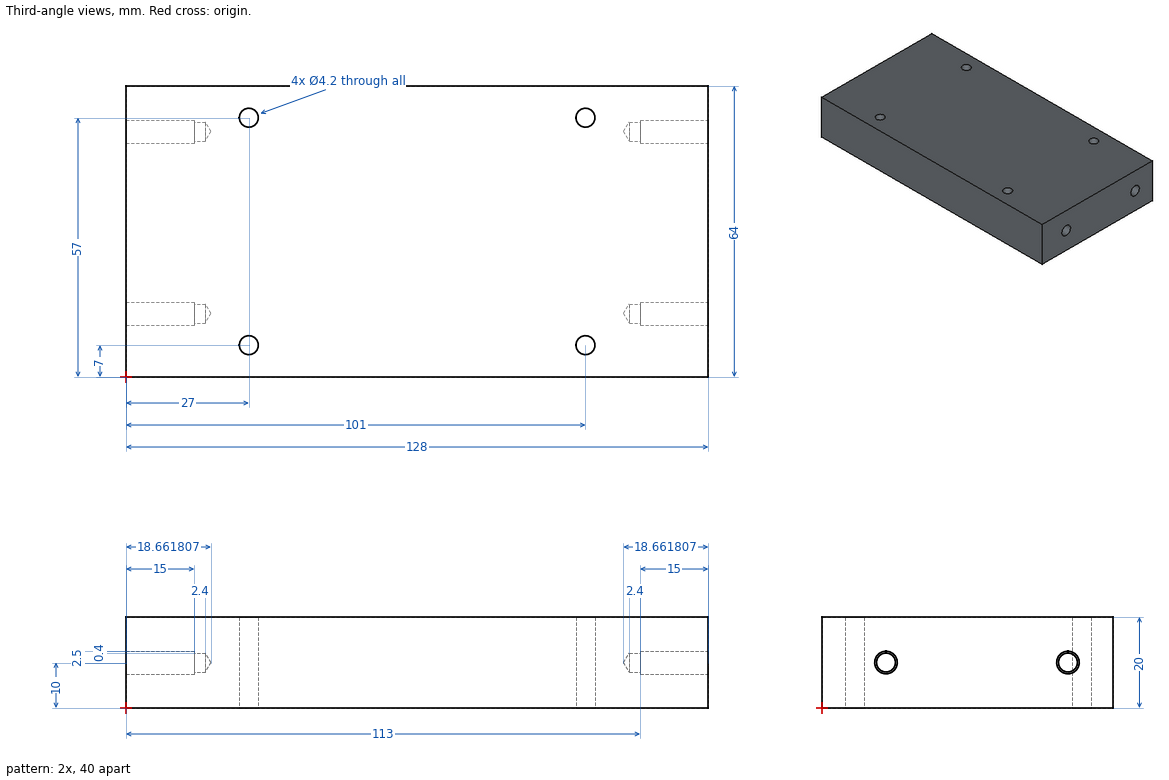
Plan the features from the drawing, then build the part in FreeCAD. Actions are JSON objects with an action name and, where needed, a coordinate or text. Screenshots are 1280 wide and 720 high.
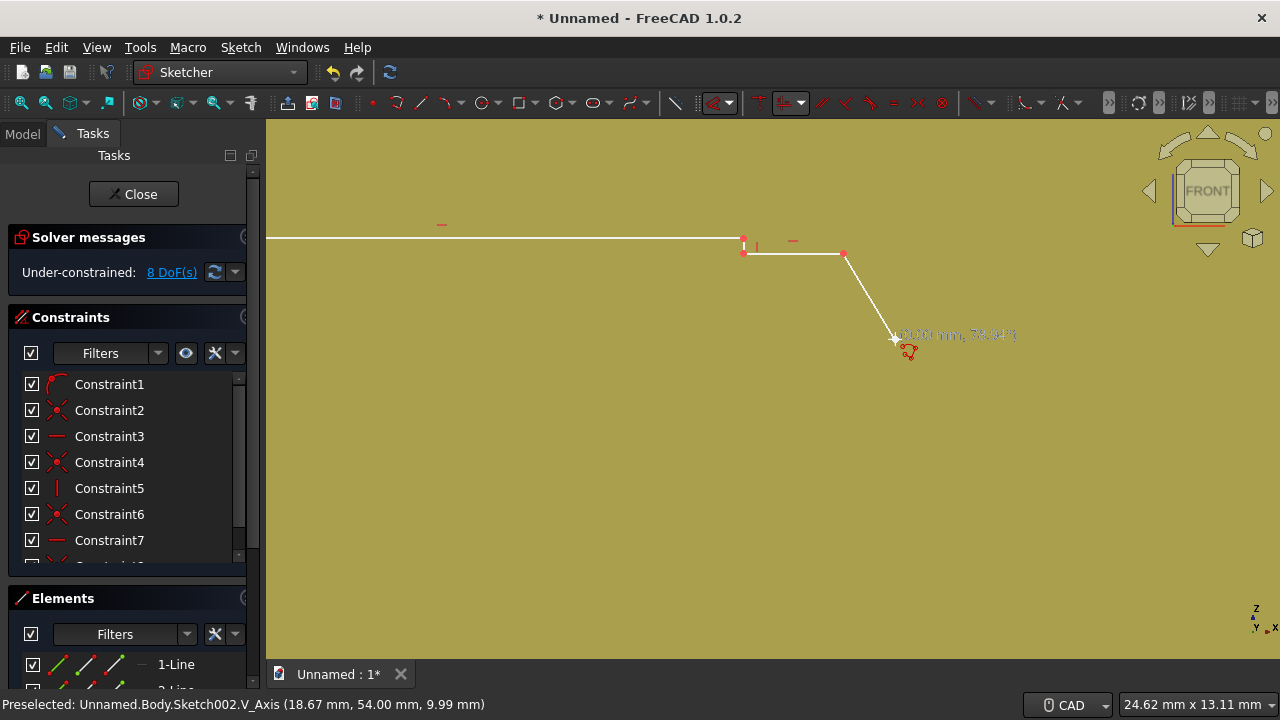
{"action": "scroll", "coordinate": [753, 262], "scroll_direction": "down", "scroll_amount": 3}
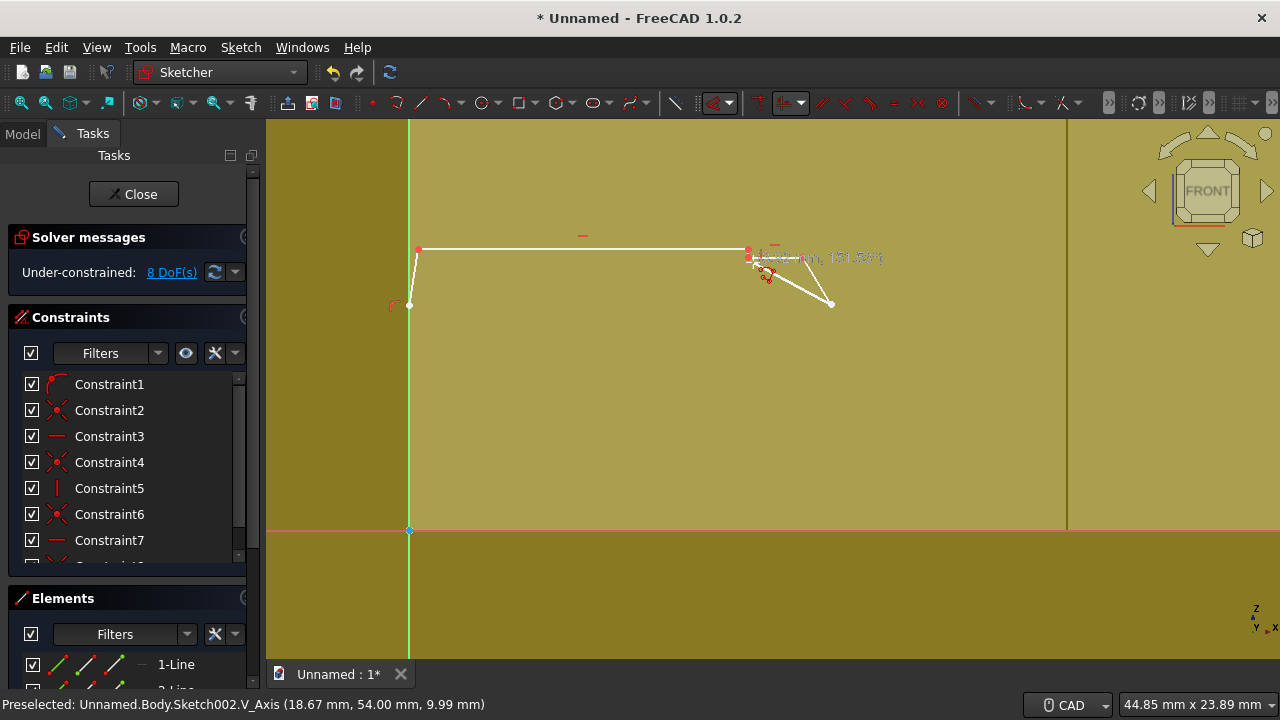
{"action": "left_click", "coordinate": [409, 305]}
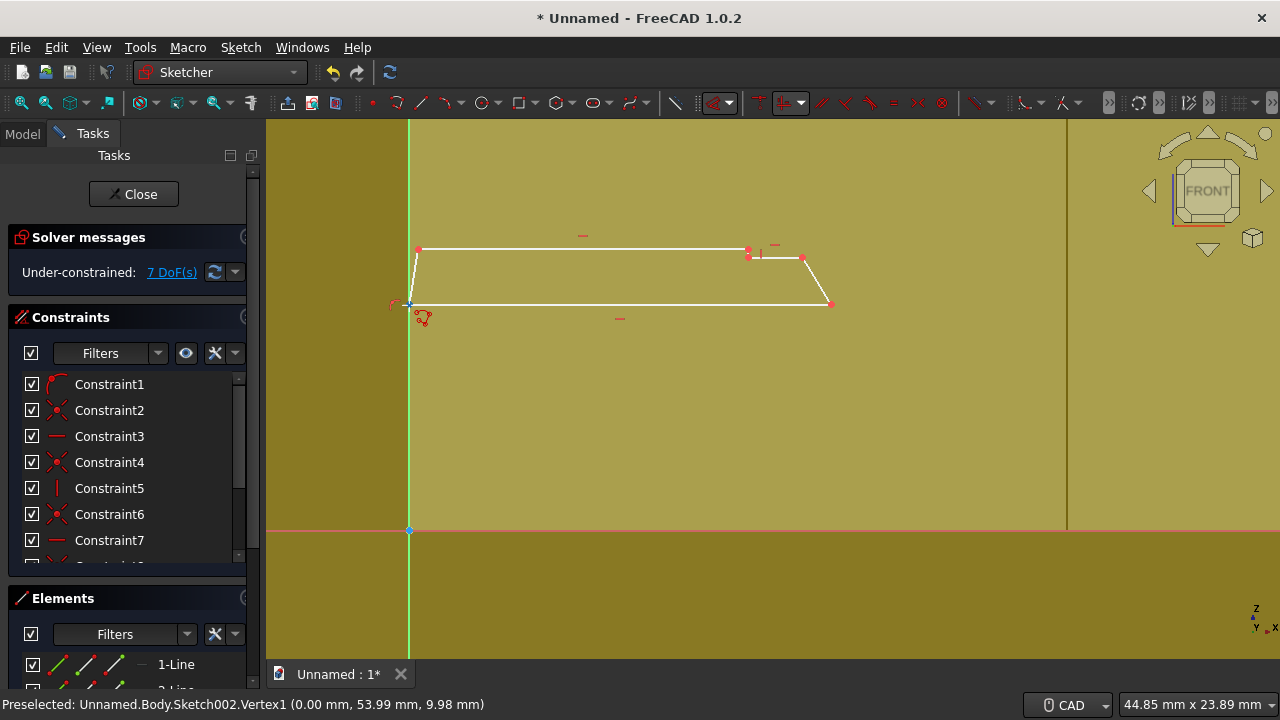
{"action": "left_click", "coordinate": [422, 104]}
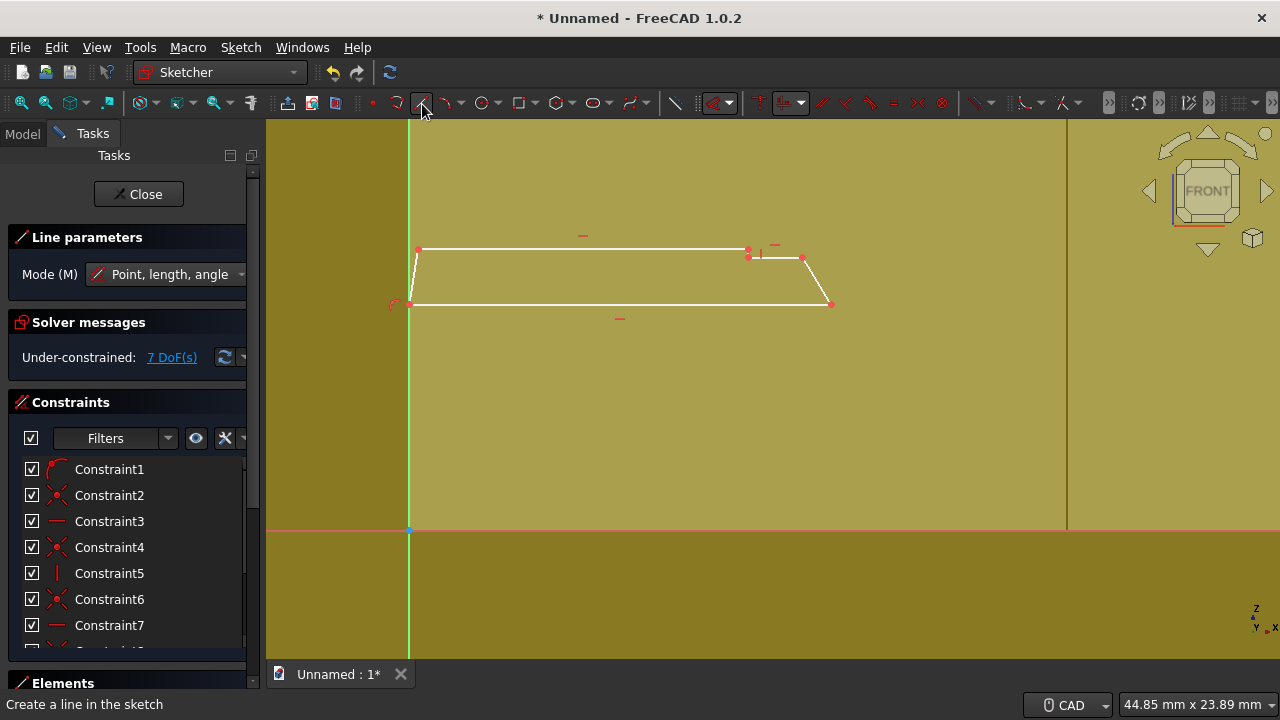
{"action": "left_click", "coordinate": [873, 305]}
{"action": "left_click", "coordinate": [1000, 305]}
{"action": "key", "text": "Escape"}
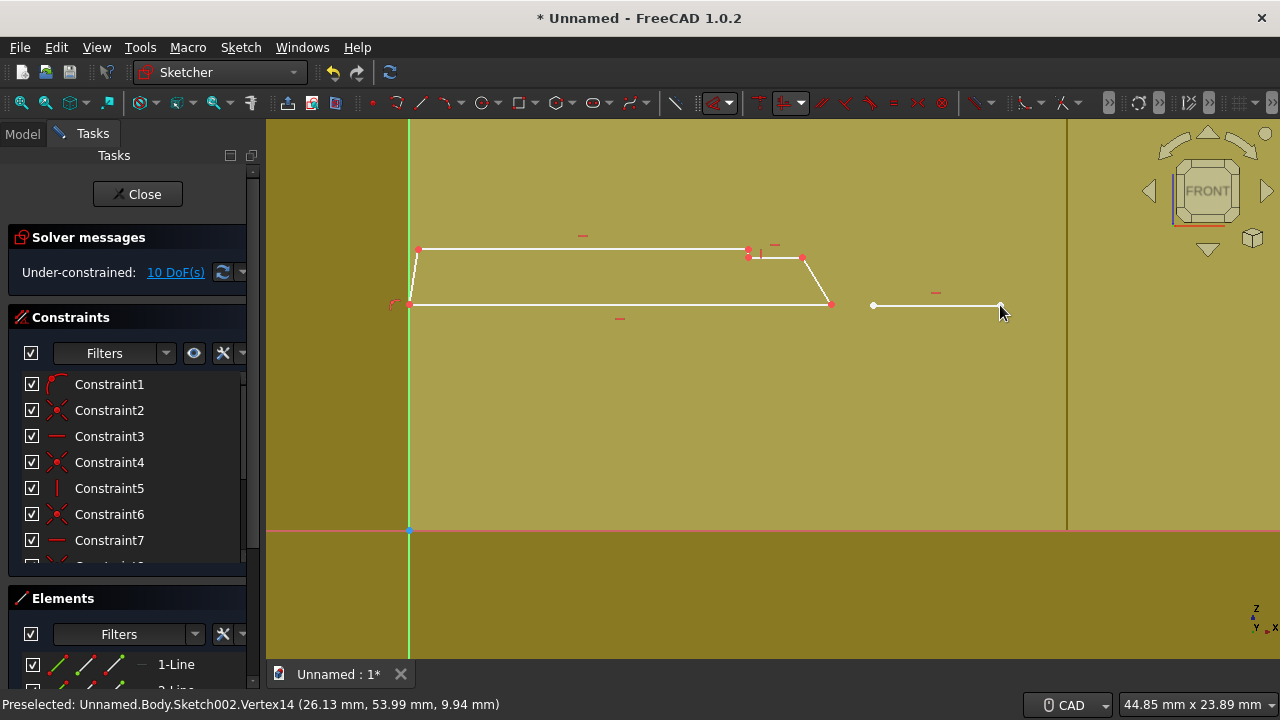
{"action": "left_click", "coordinate": [911, 306]}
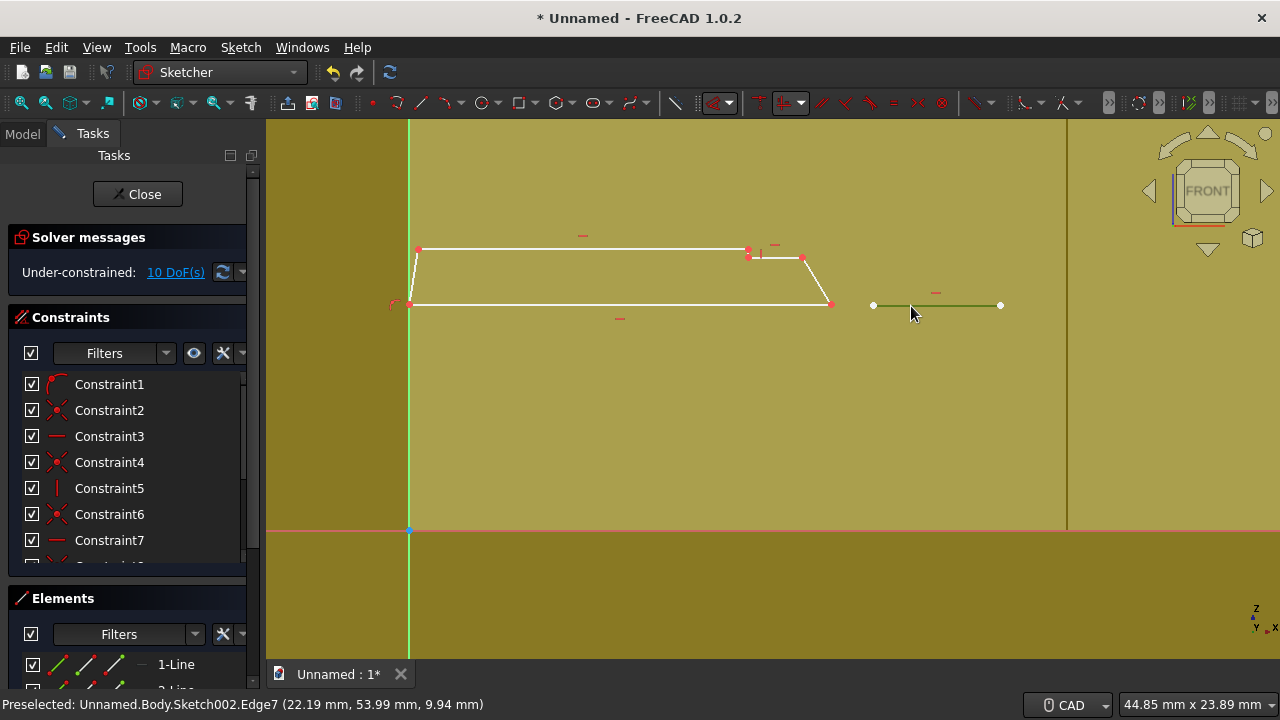
{"action": "left_click", "coordinate": [676, 104]}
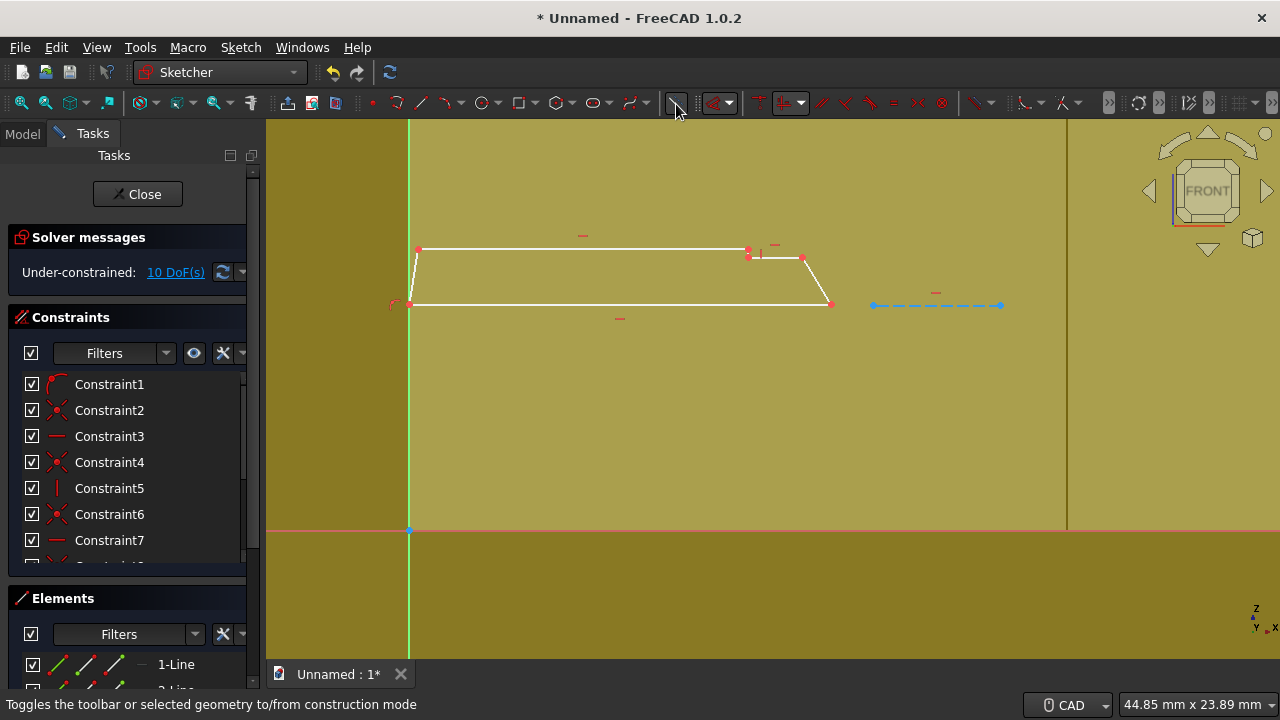
{"action": "left_click", "coordinate": [412, 288]}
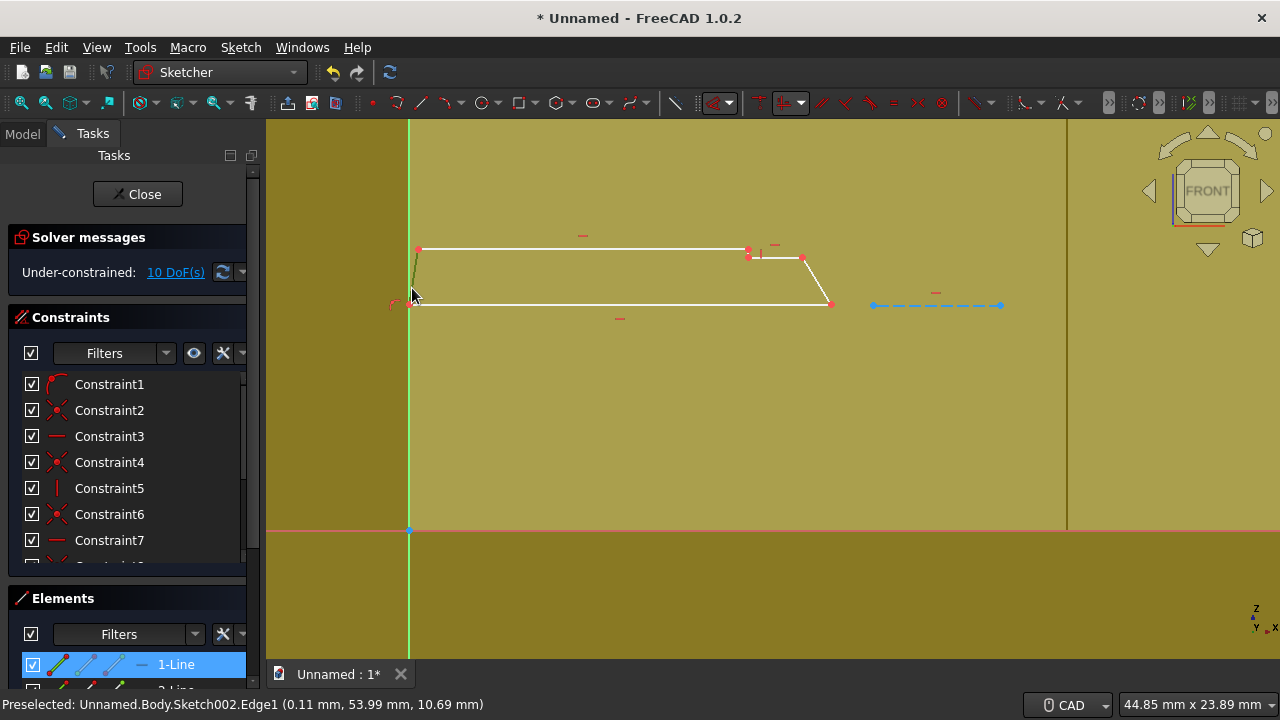
{"action": "key", "text": "v"}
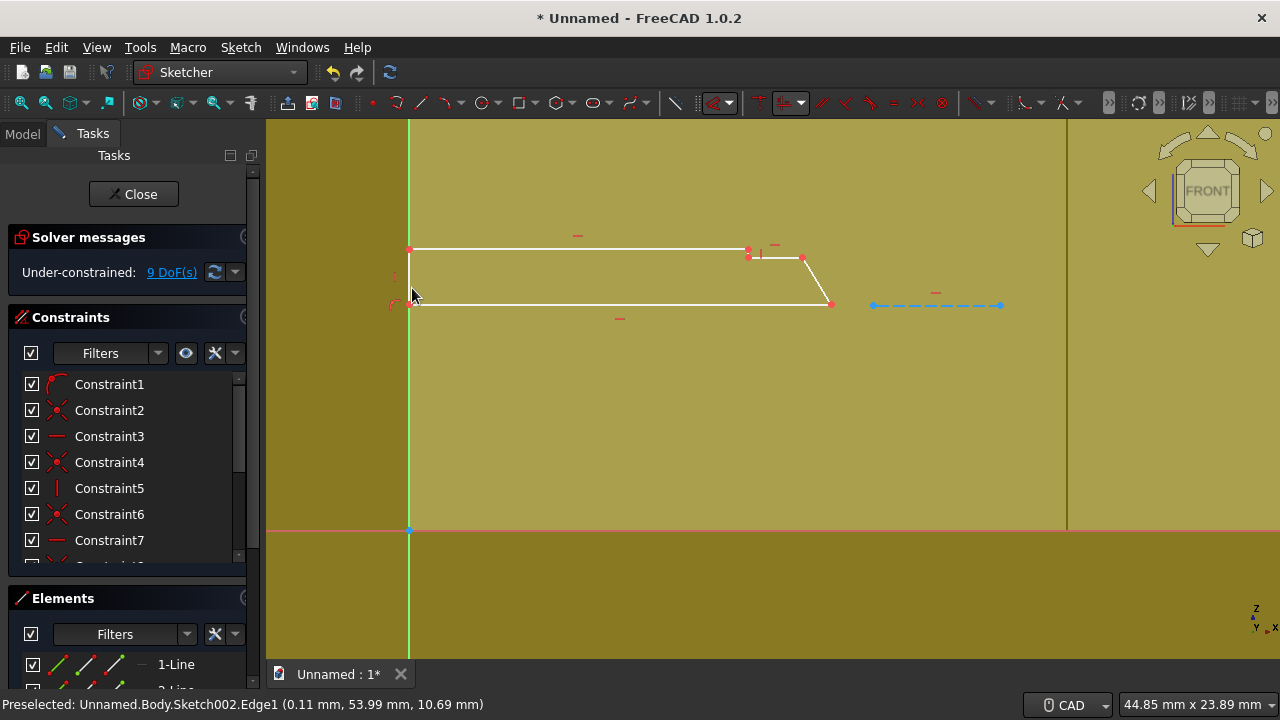
{"action": "left_click", "coordinate": [511, 249]}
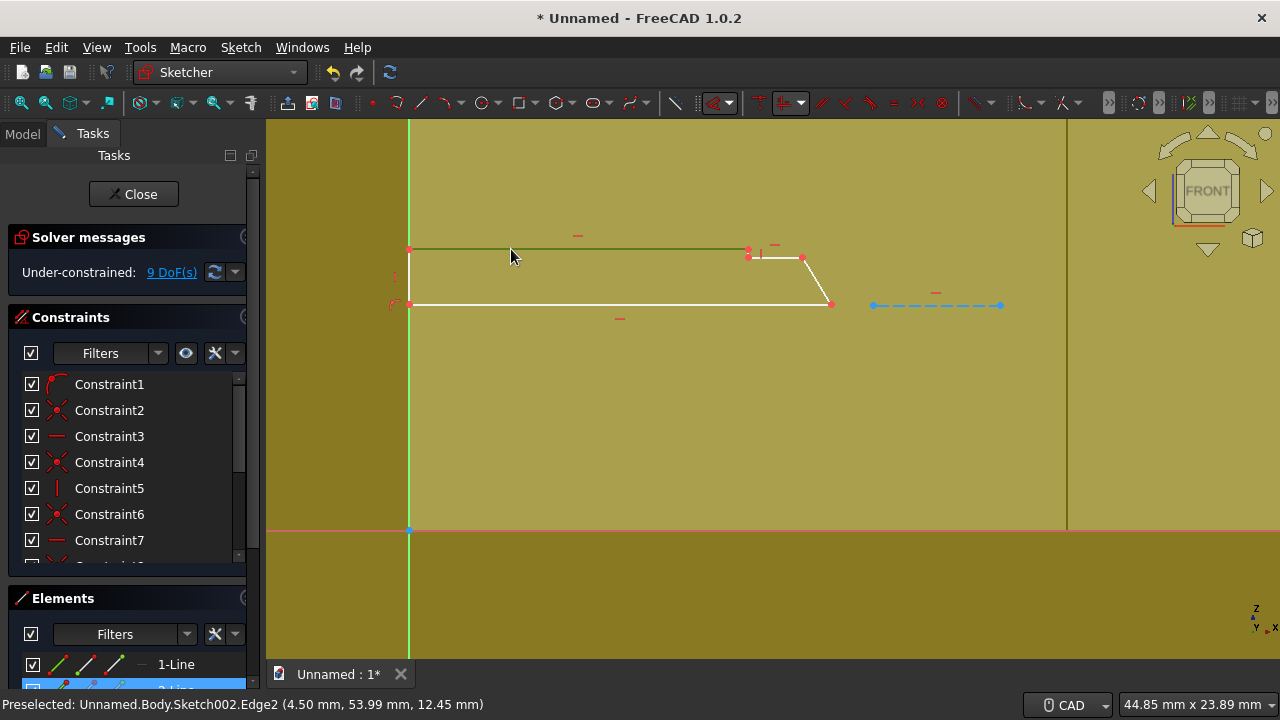
{"action": "left_click", "coordinate": [732, 104]}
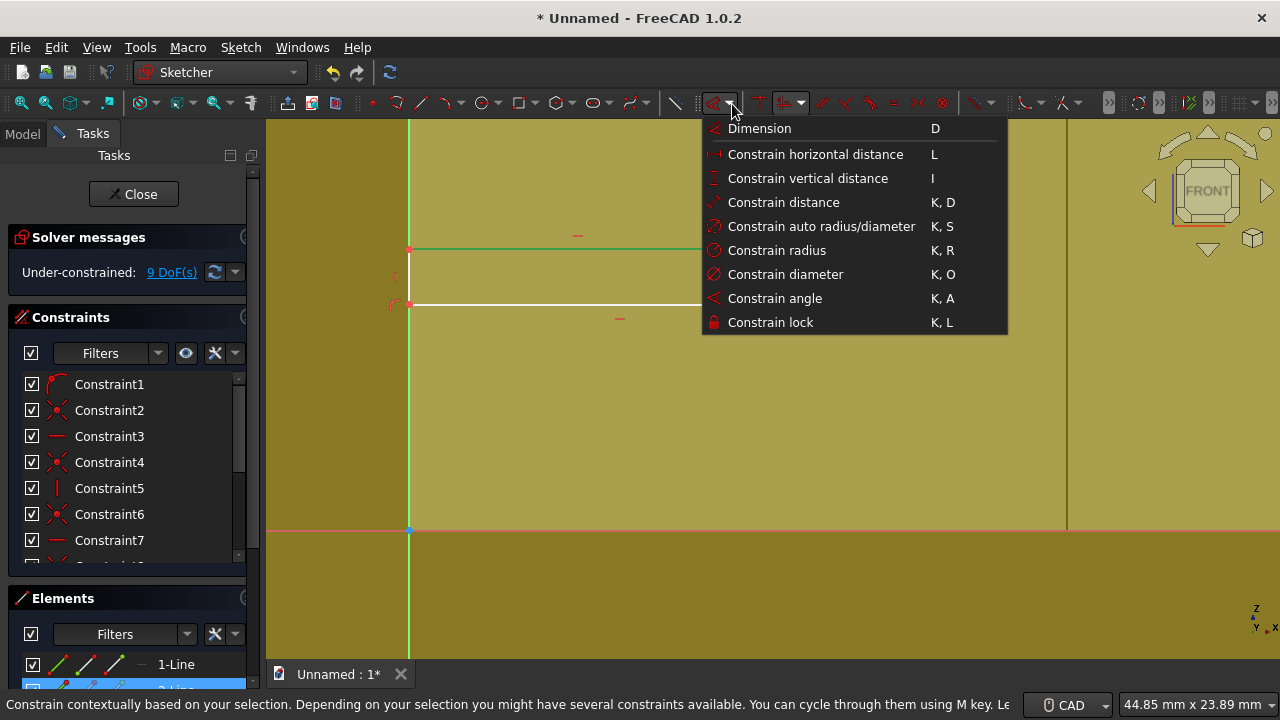
{"action": "left_click", "coordinate": [855, 154]}